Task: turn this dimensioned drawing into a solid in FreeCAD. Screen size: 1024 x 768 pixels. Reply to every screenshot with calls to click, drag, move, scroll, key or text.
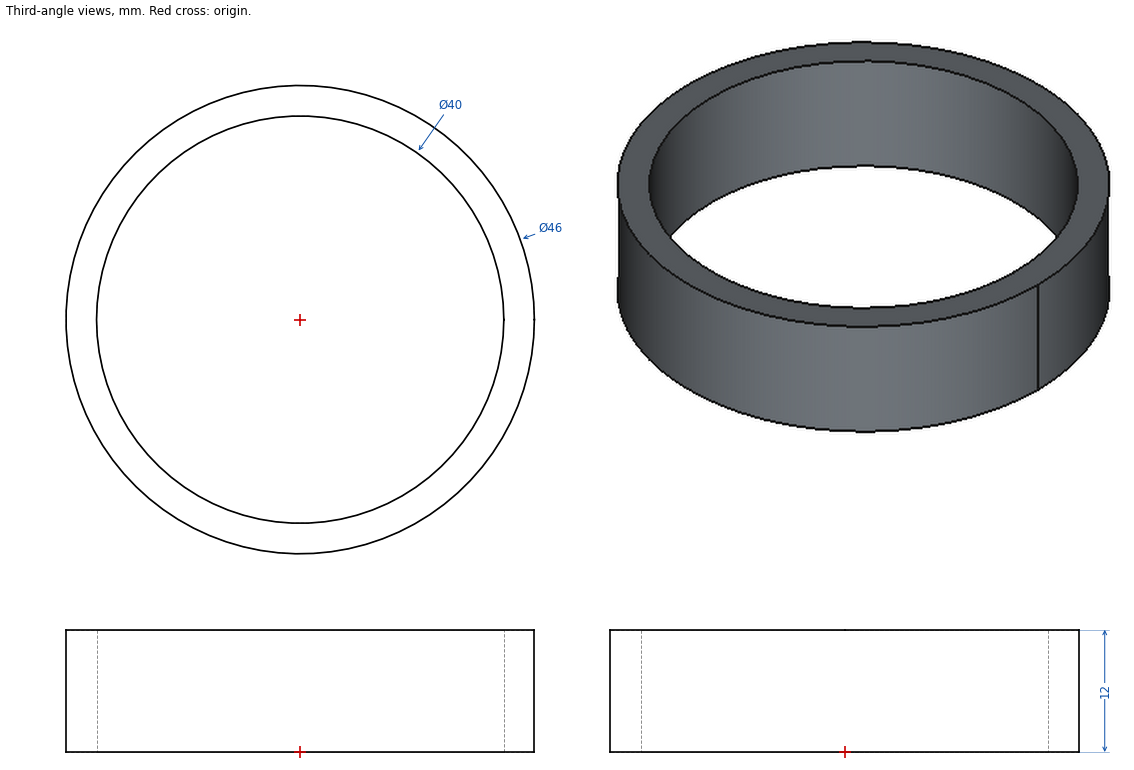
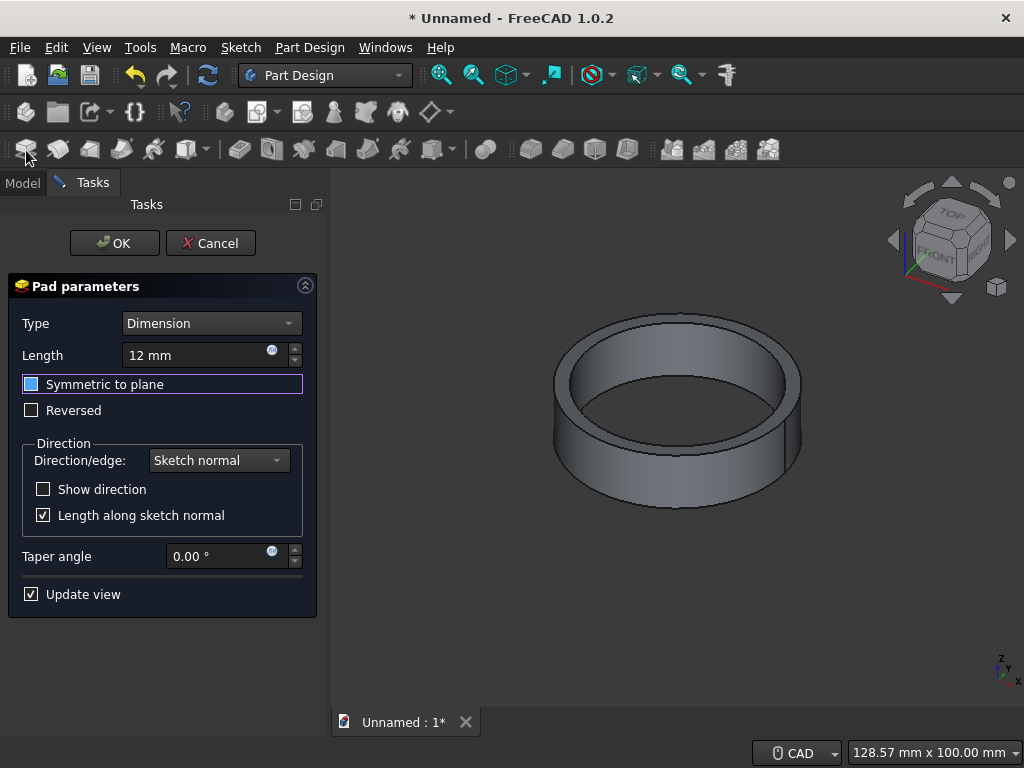
click(115, 243)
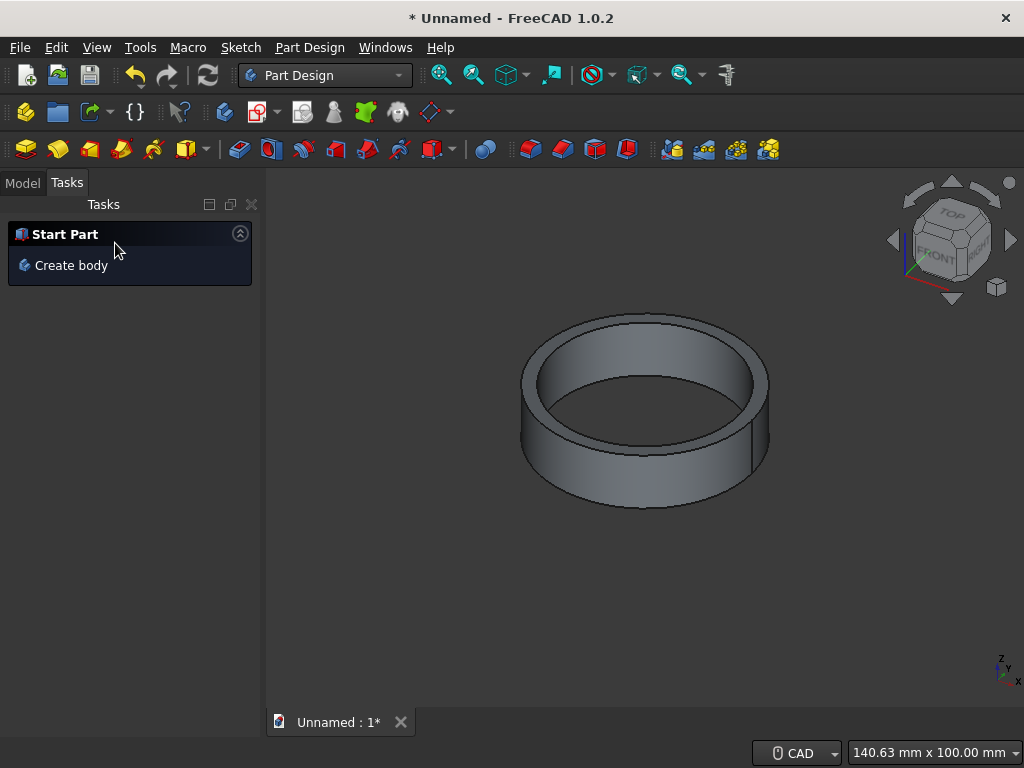
key(0)